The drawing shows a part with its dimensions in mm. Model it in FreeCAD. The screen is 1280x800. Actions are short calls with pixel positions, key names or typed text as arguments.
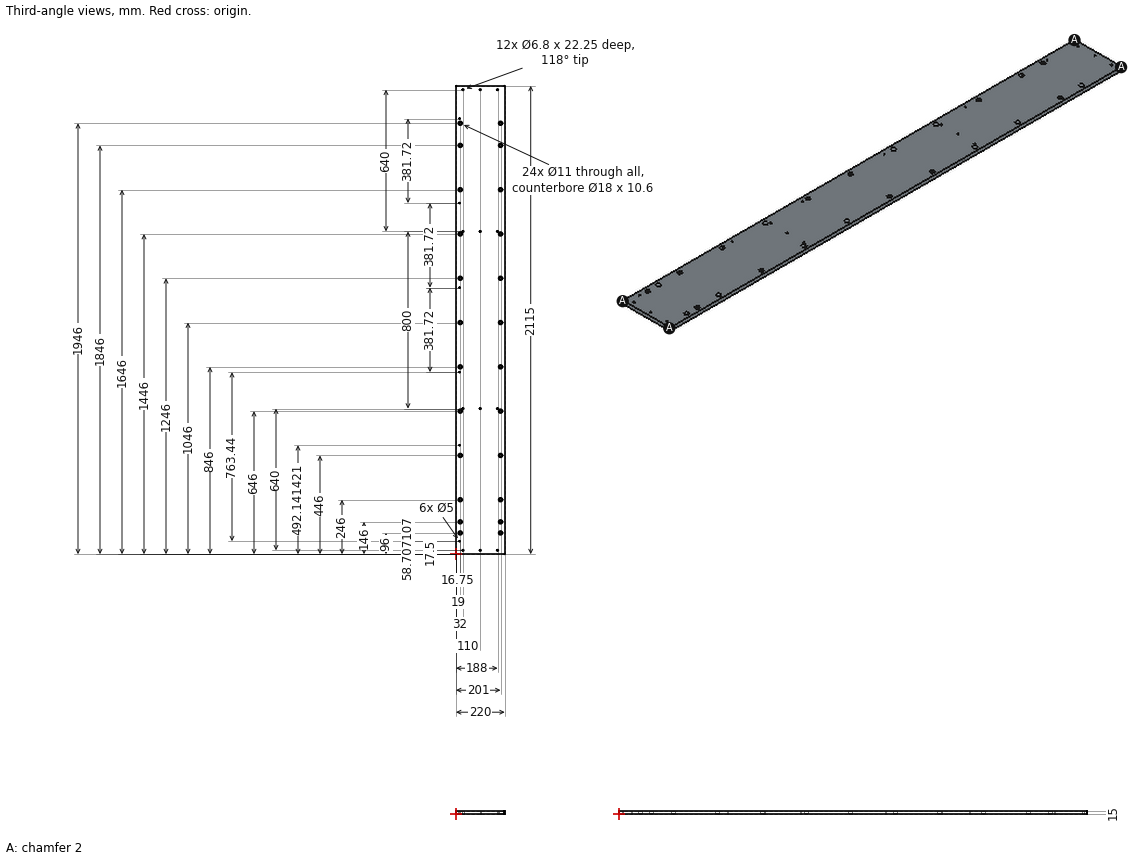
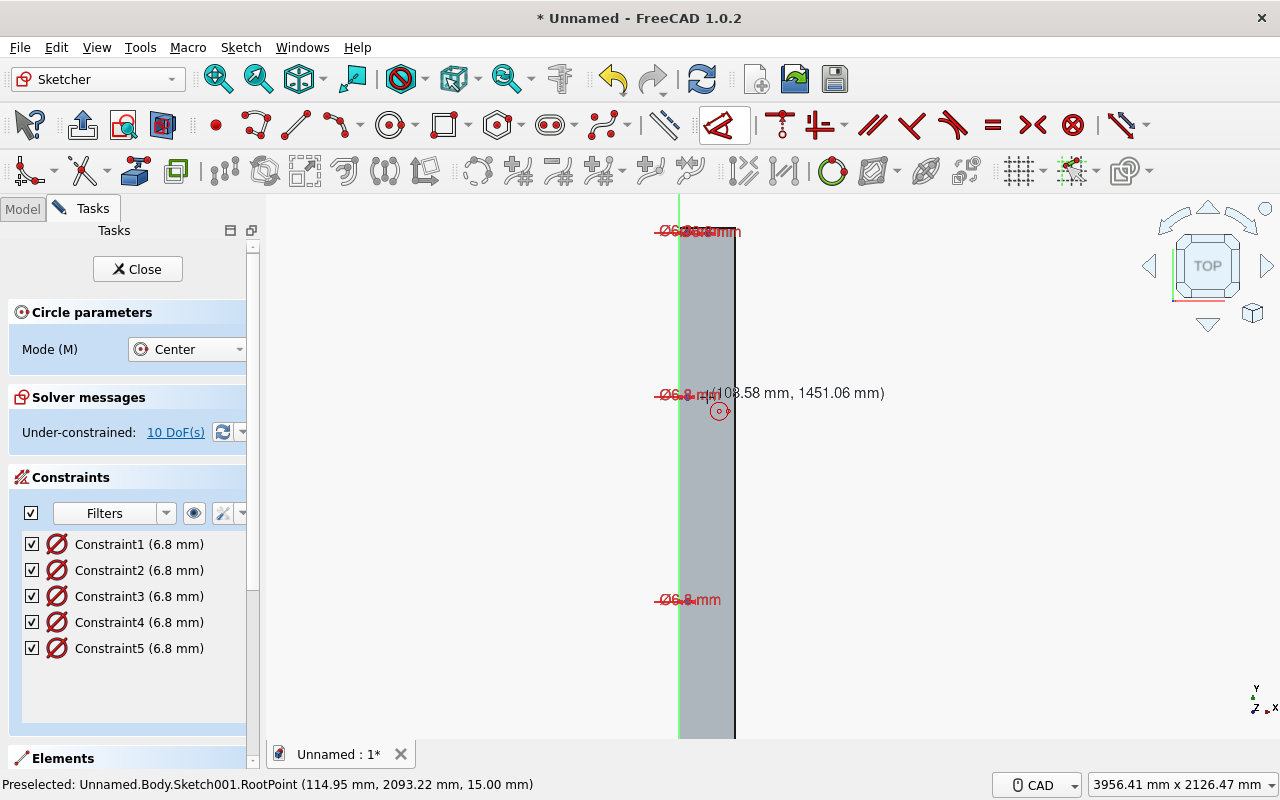
click(707, 397)
move(708, 396)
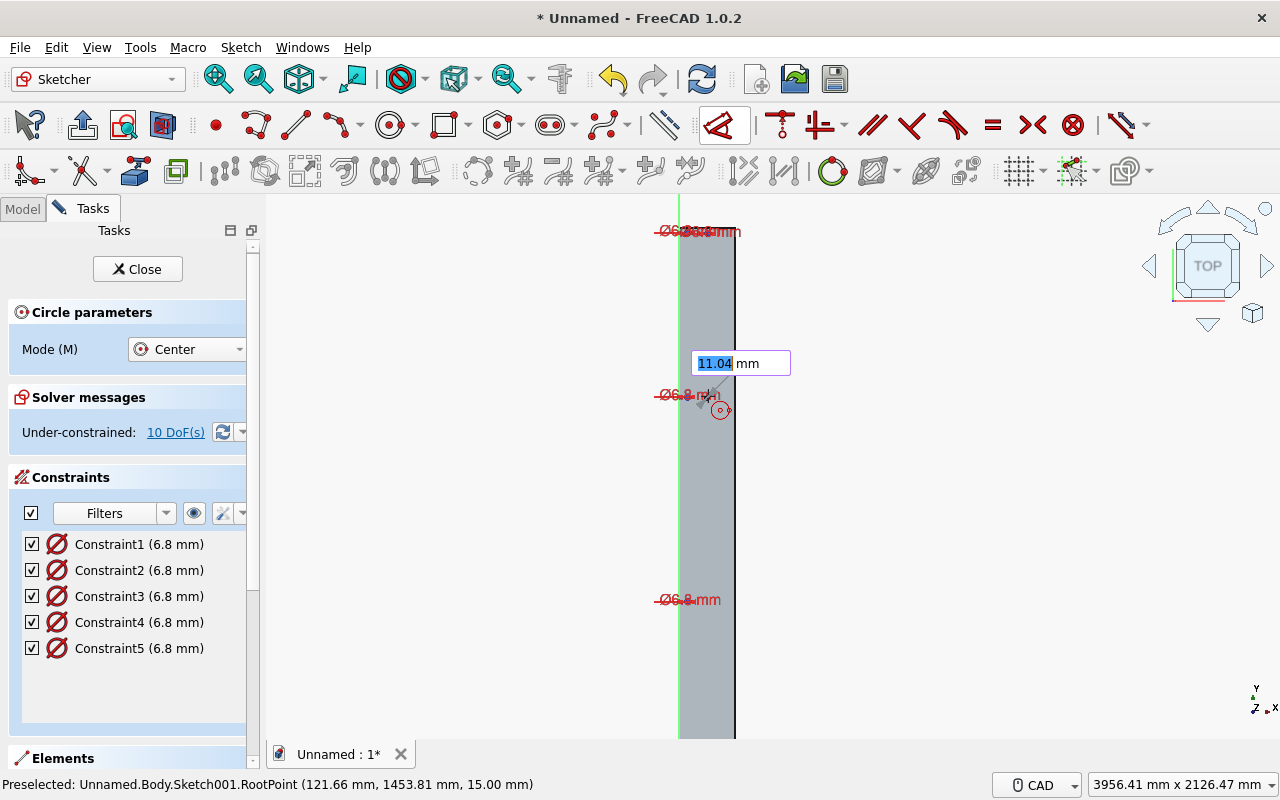
text(6.8)
key(Return)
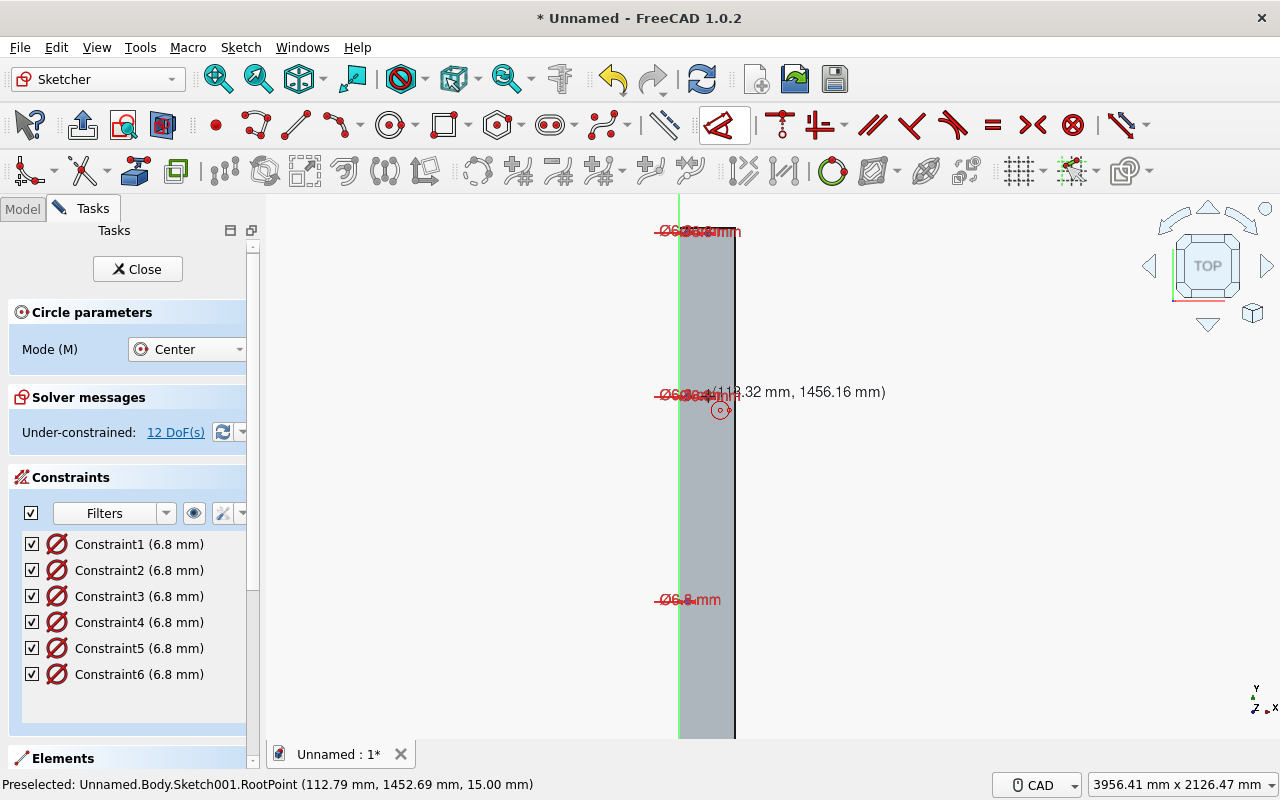
scroll(707, 602, up, 17)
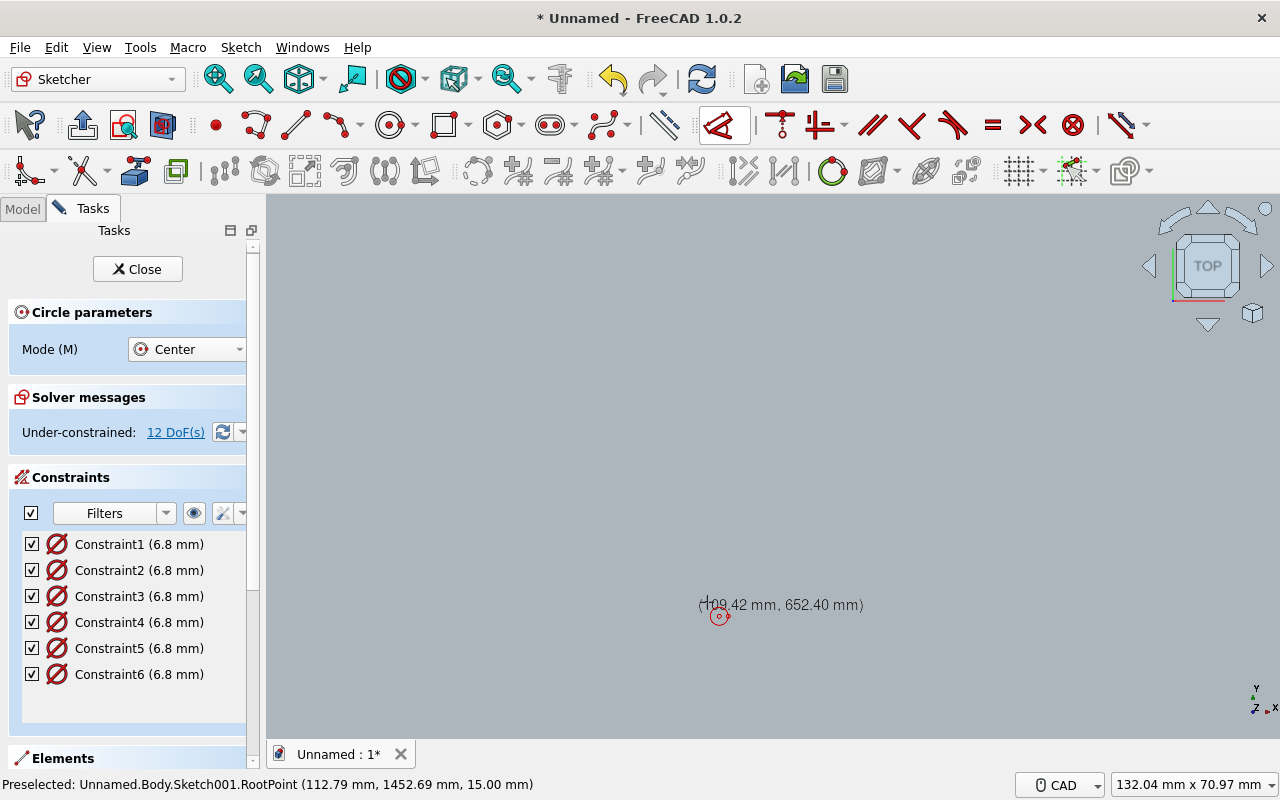
scroll(704, 466, down, 15)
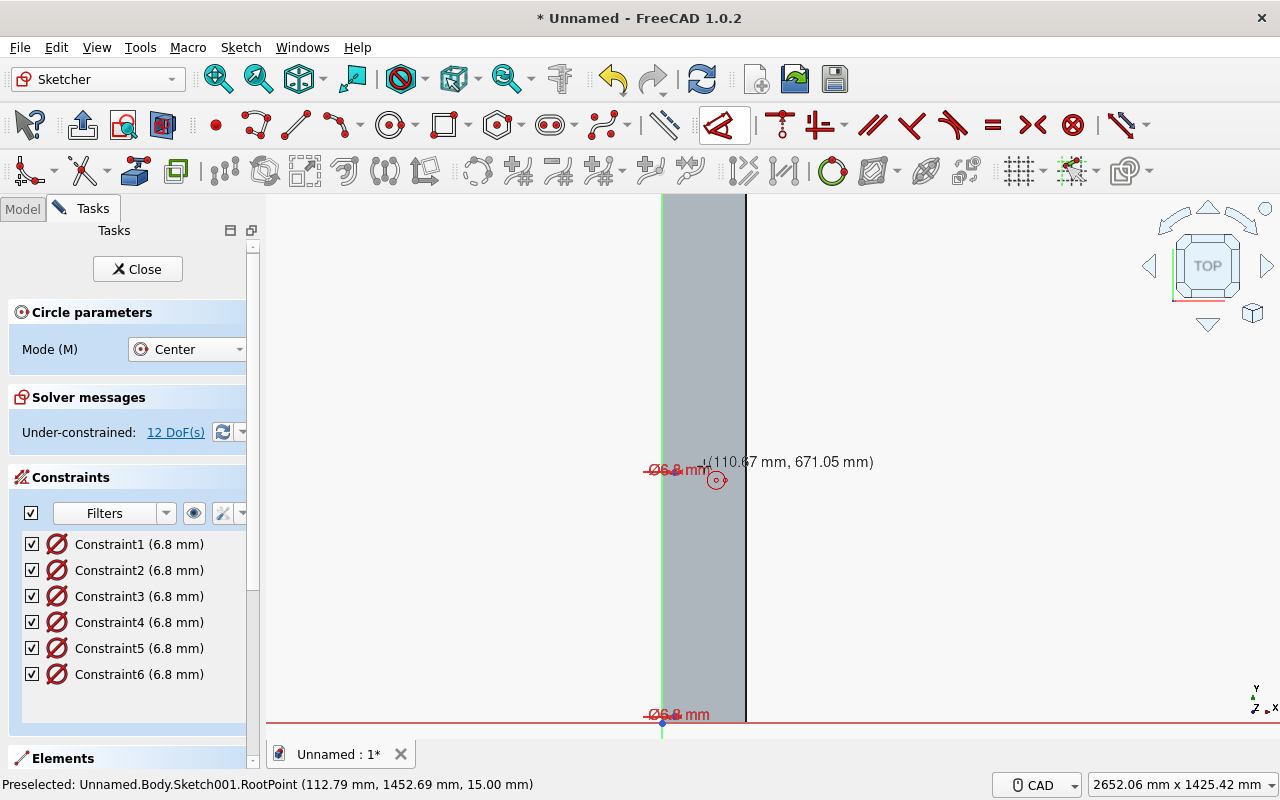
scroll(709, 585, down, 4)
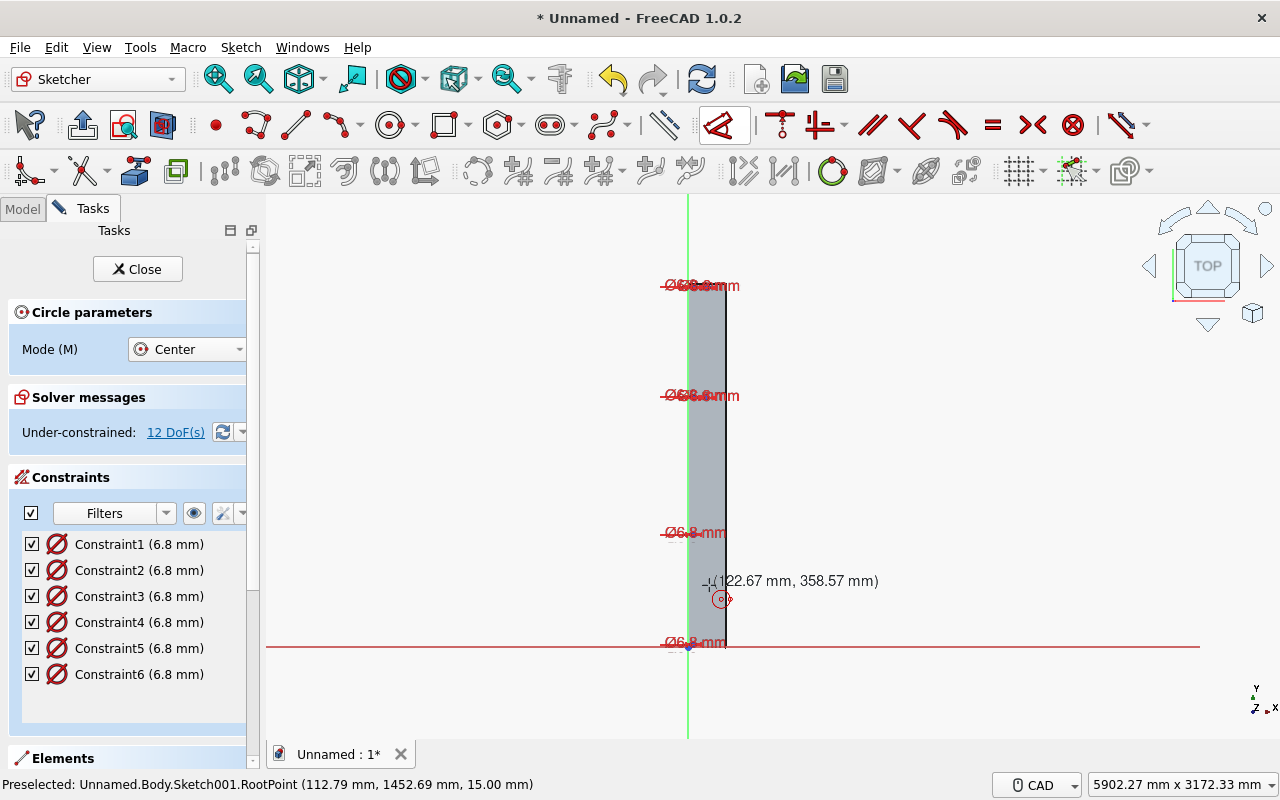
scroll(707, 534, up, 2)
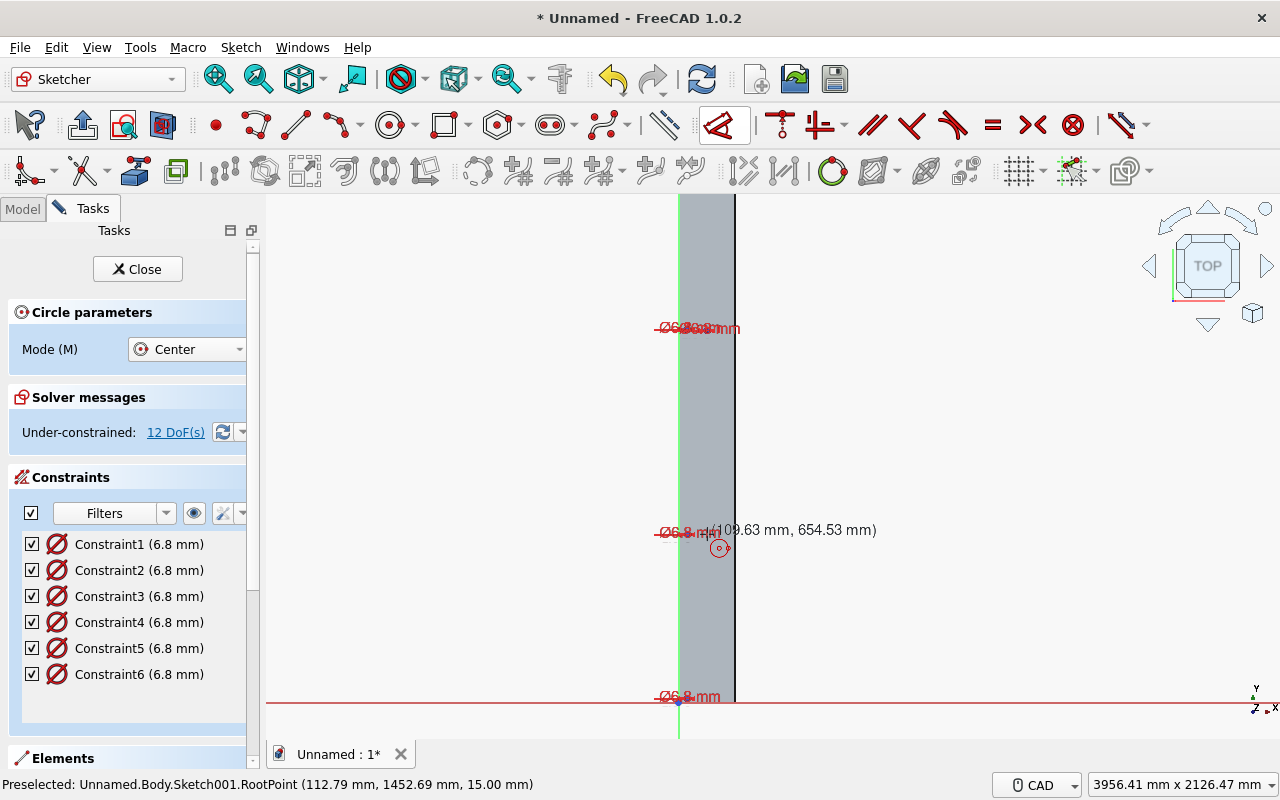
click(707, 534)
move(707, 534)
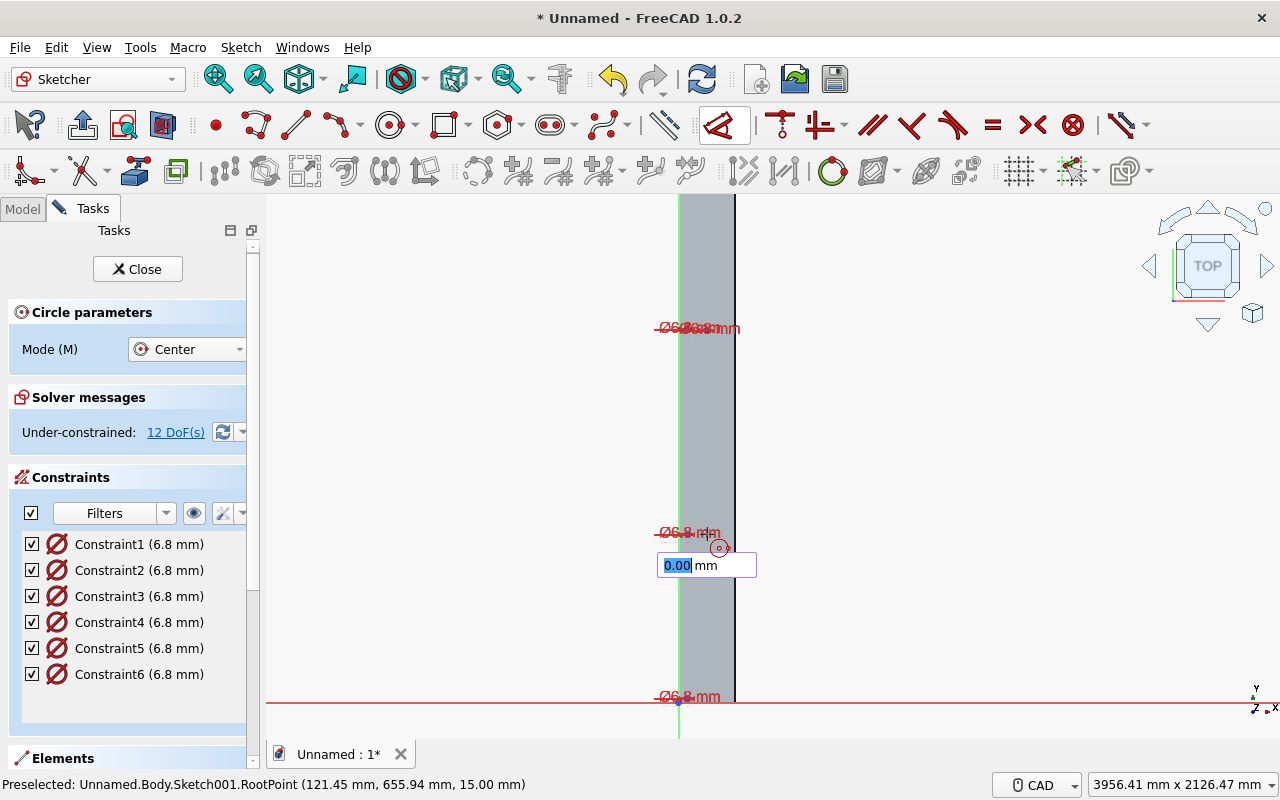
text(6.8)
key(Return)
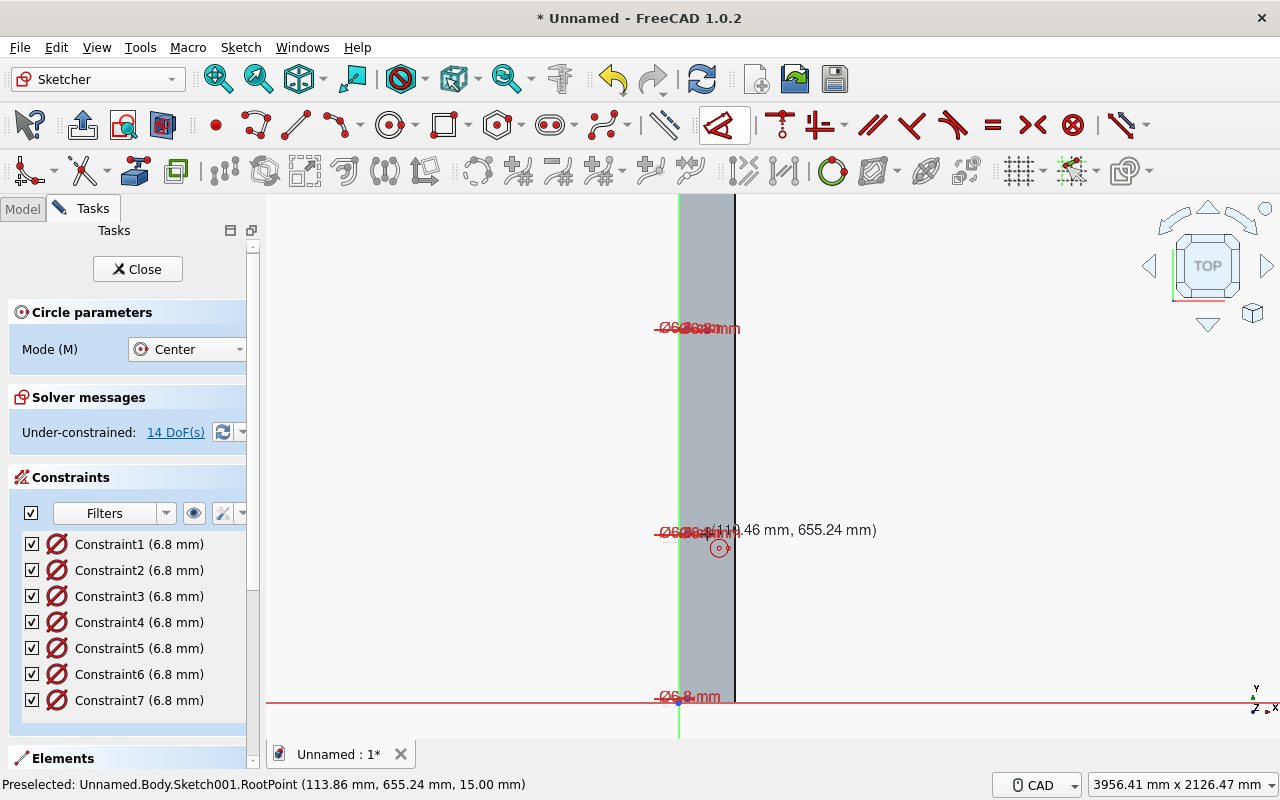
scroll(707, 698, up, 17)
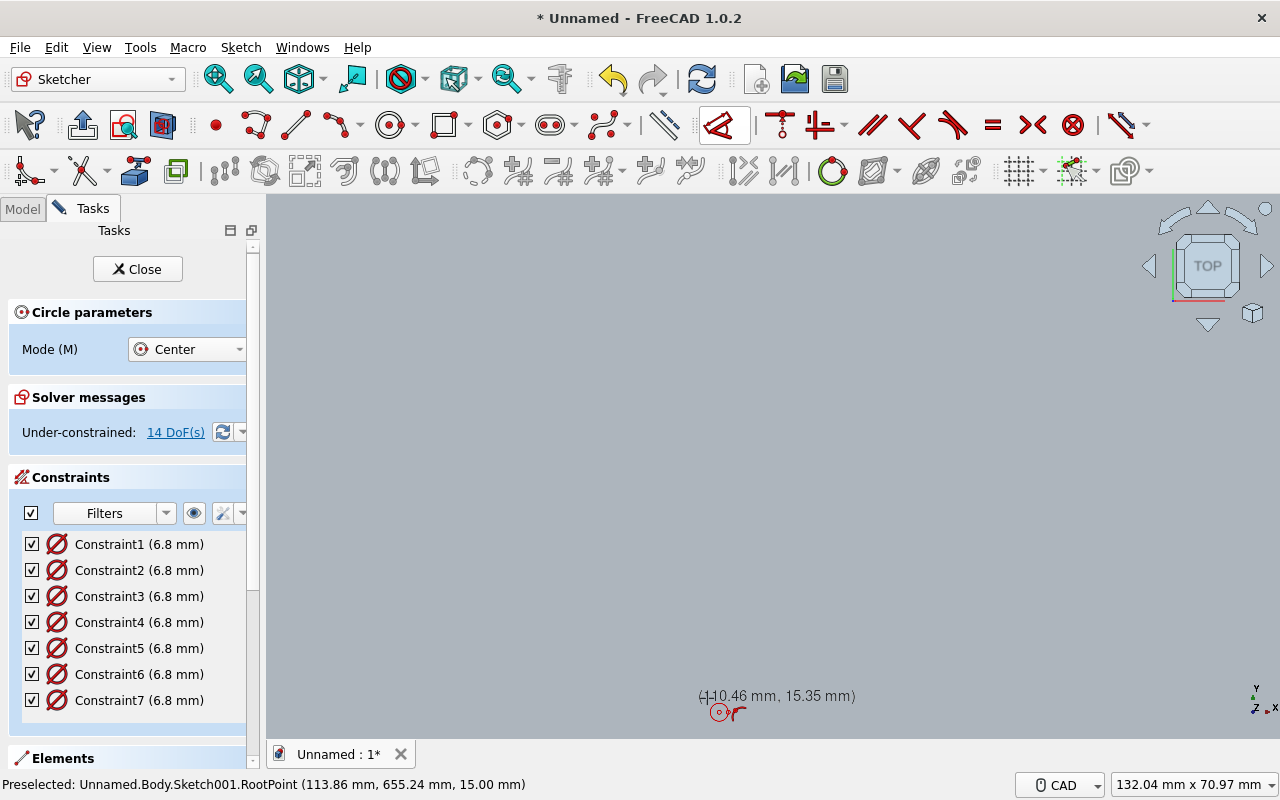
scroll(704, 466, down, 15)